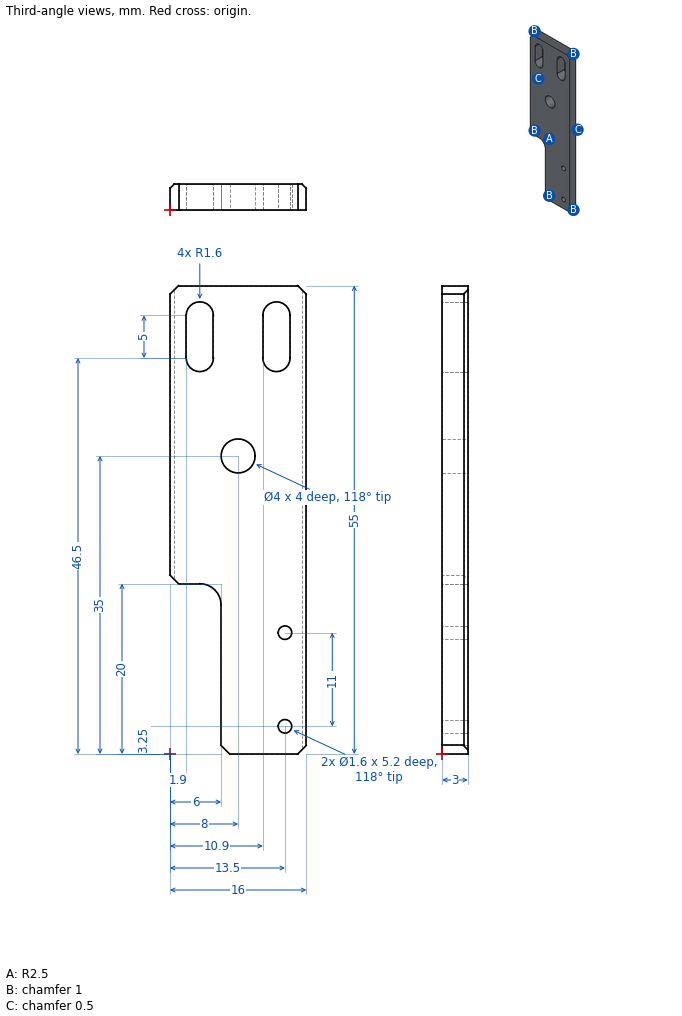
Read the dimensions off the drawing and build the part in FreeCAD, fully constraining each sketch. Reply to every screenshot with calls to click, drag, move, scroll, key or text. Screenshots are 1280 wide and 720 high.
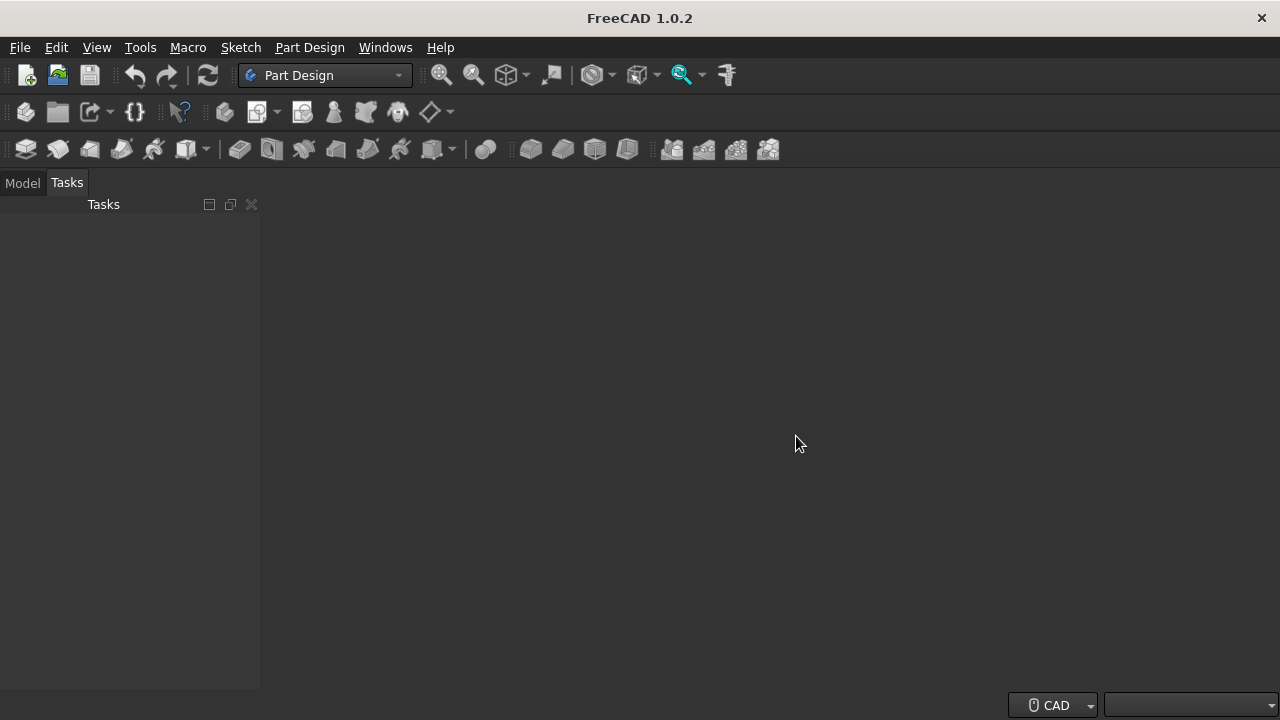
click(26, 76)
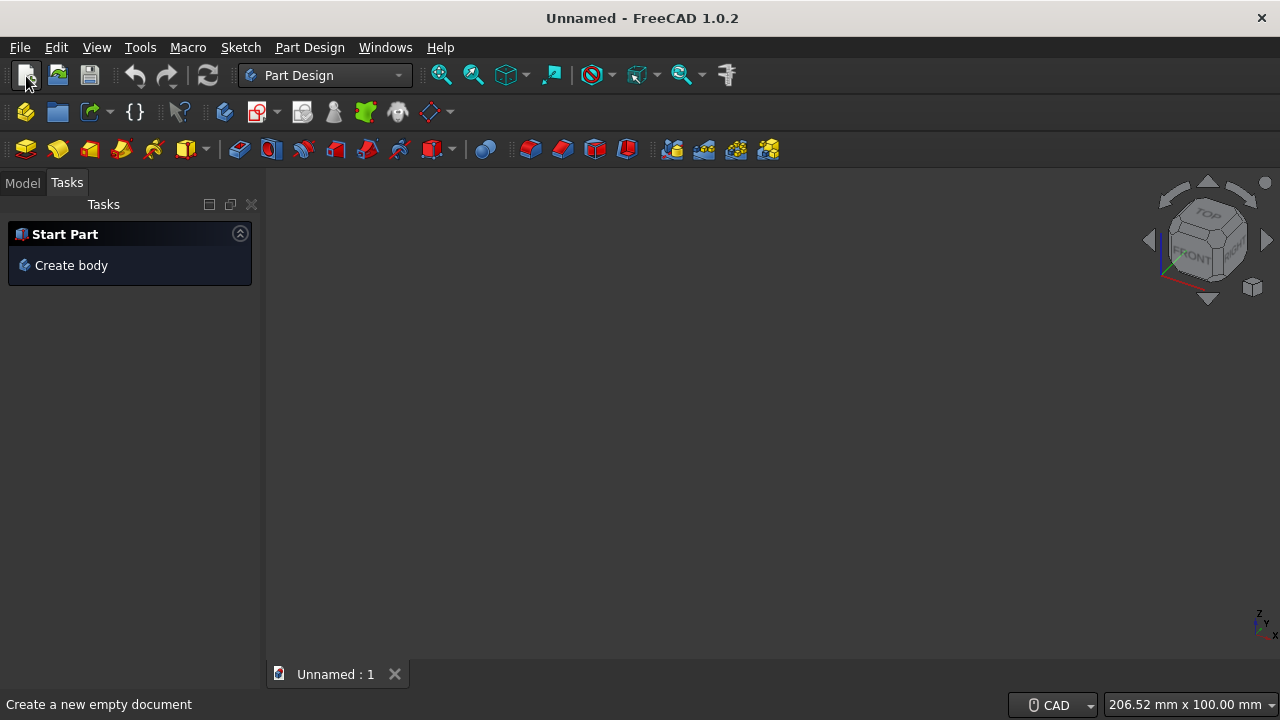
click(258, 112)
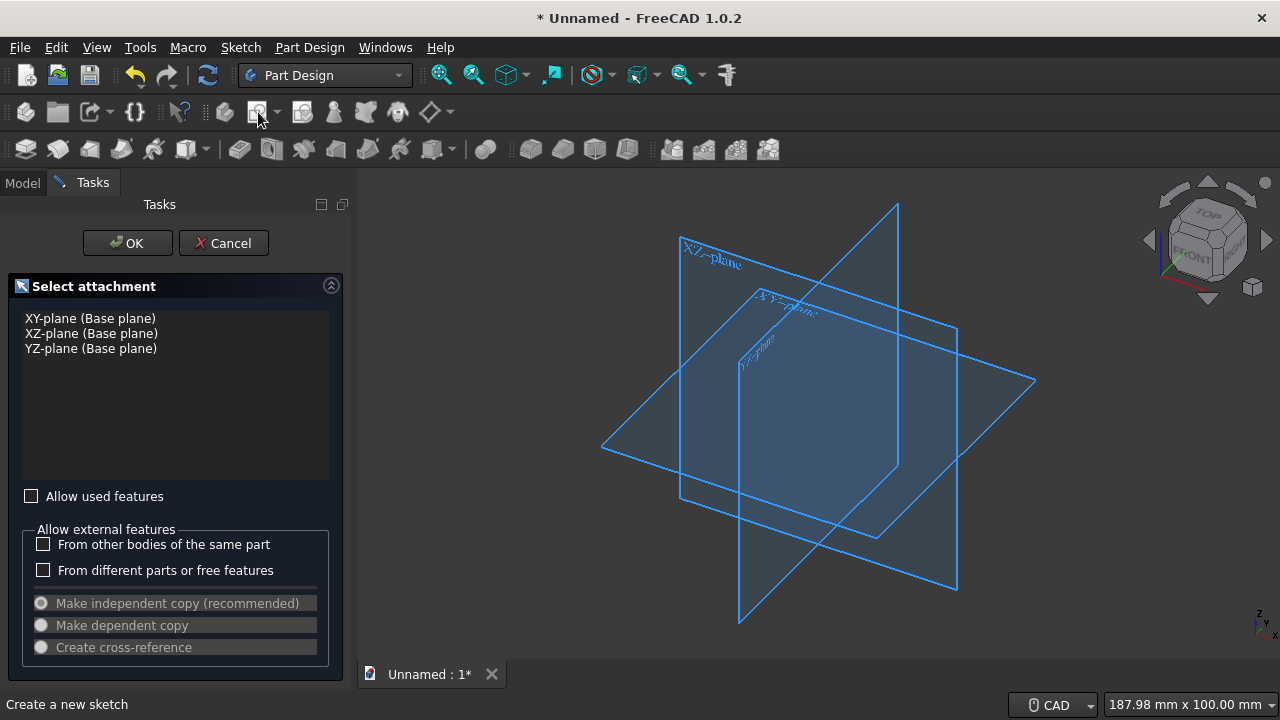
click(82, 334)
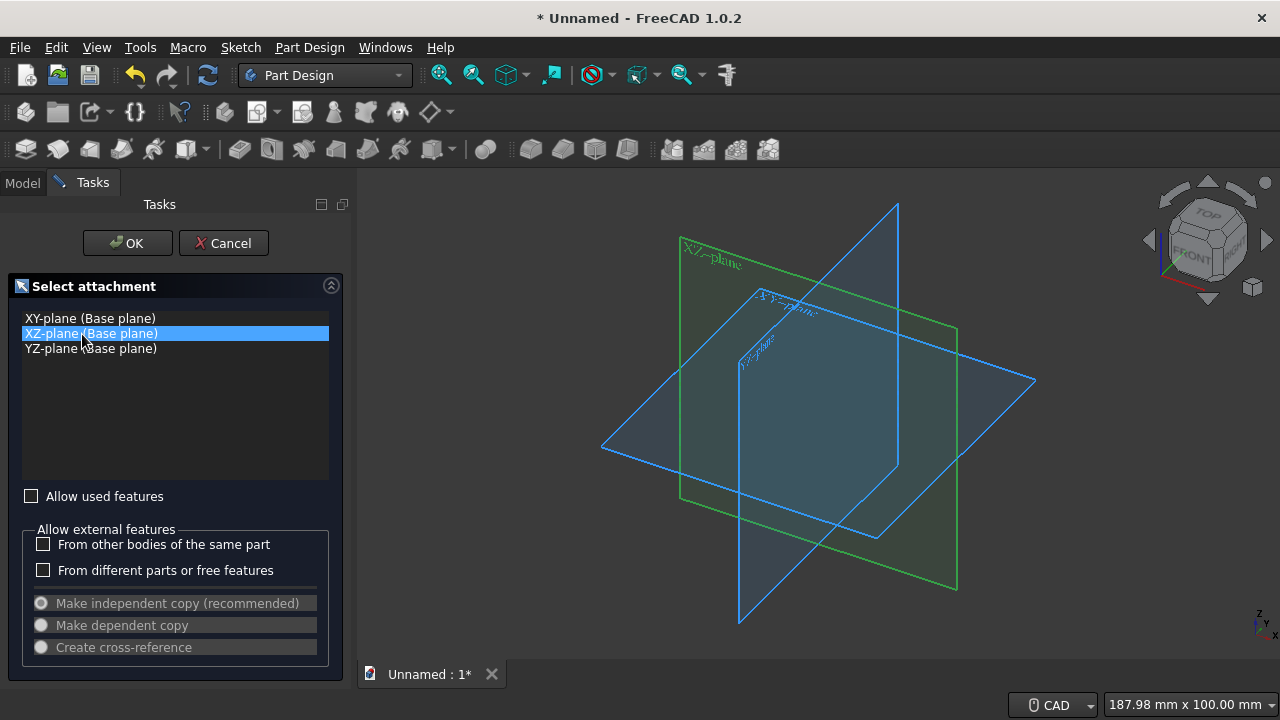
click(128, 243)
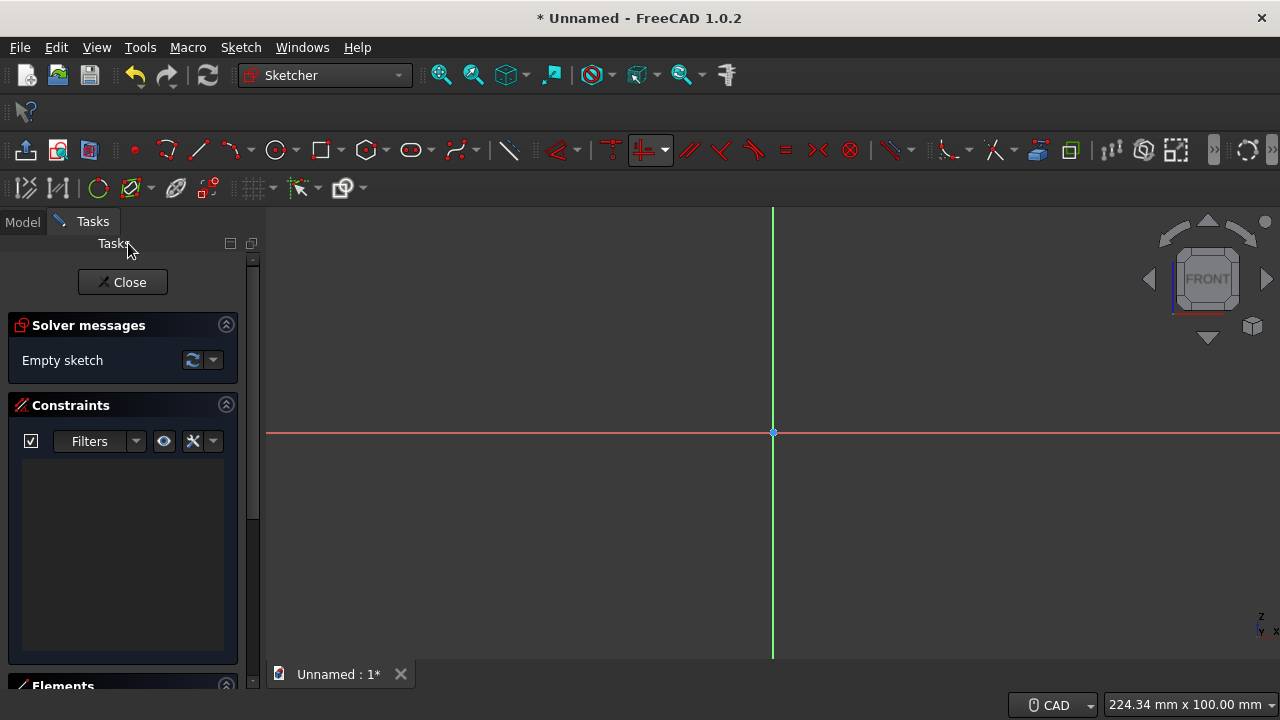
scroll(294, 631, down, 1)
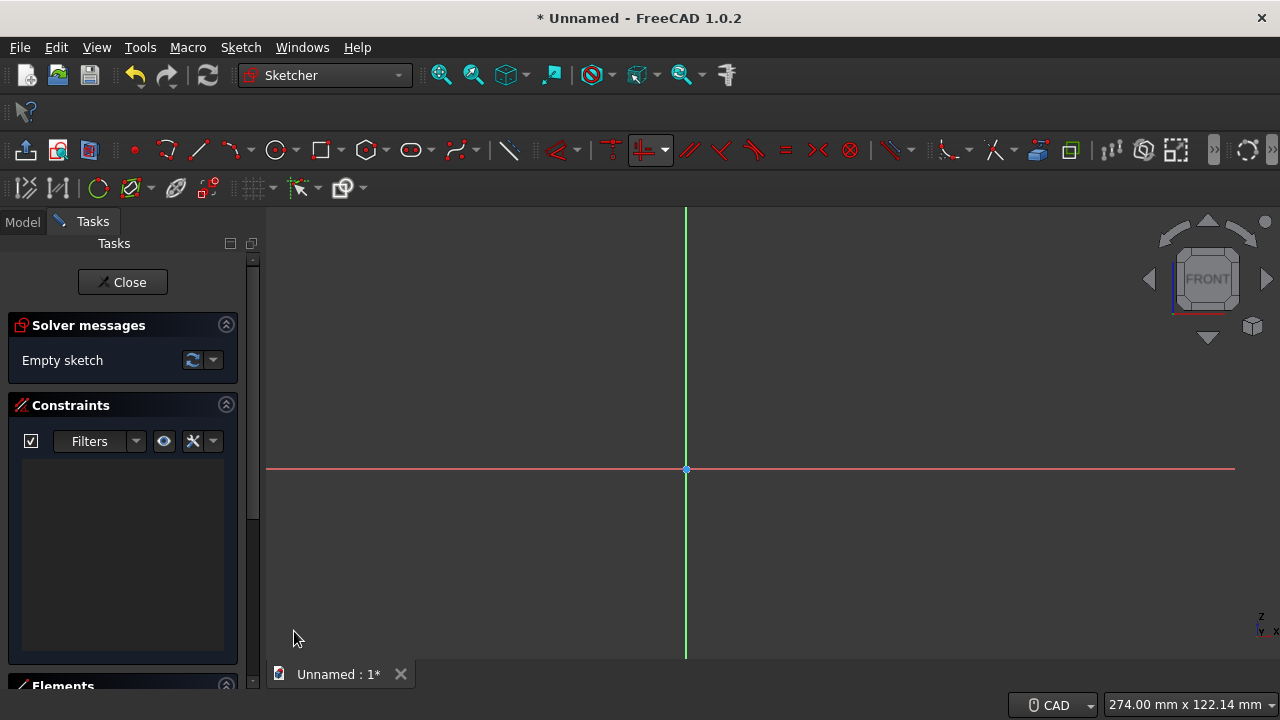
scroll(739, 235, up, 2)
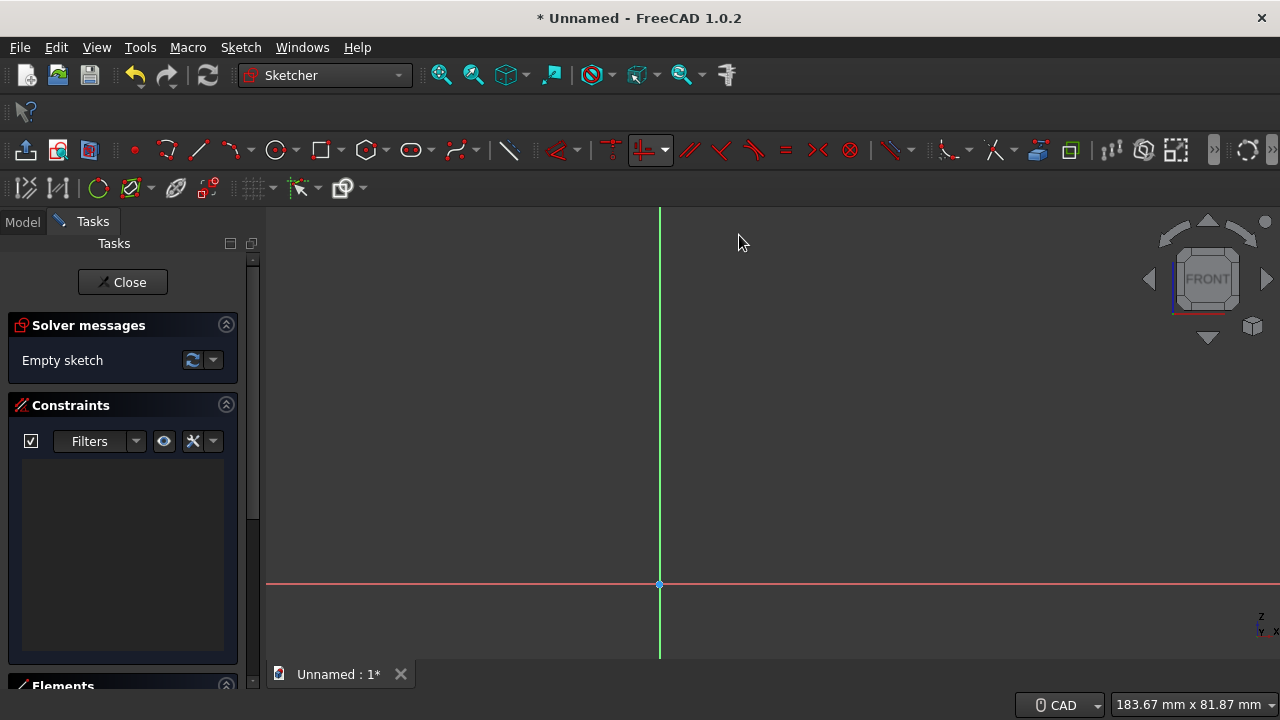
click(322, 150)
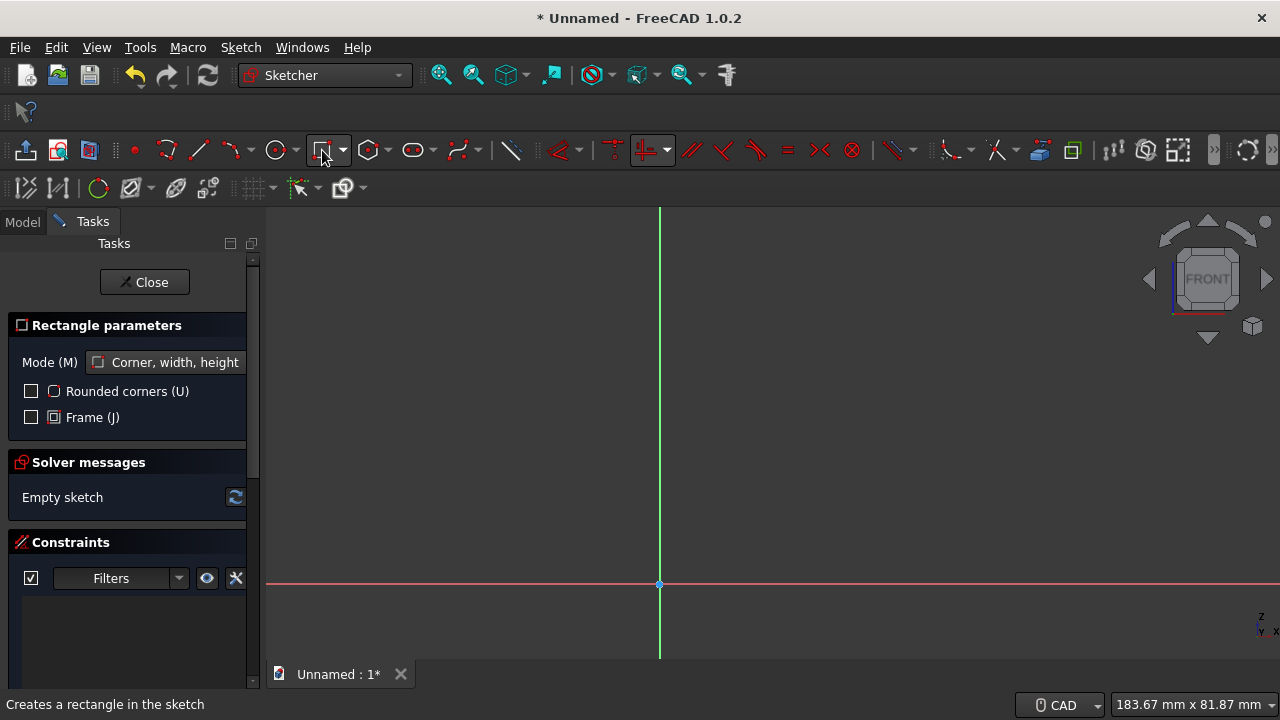
click(660, 584)
move(748, 281)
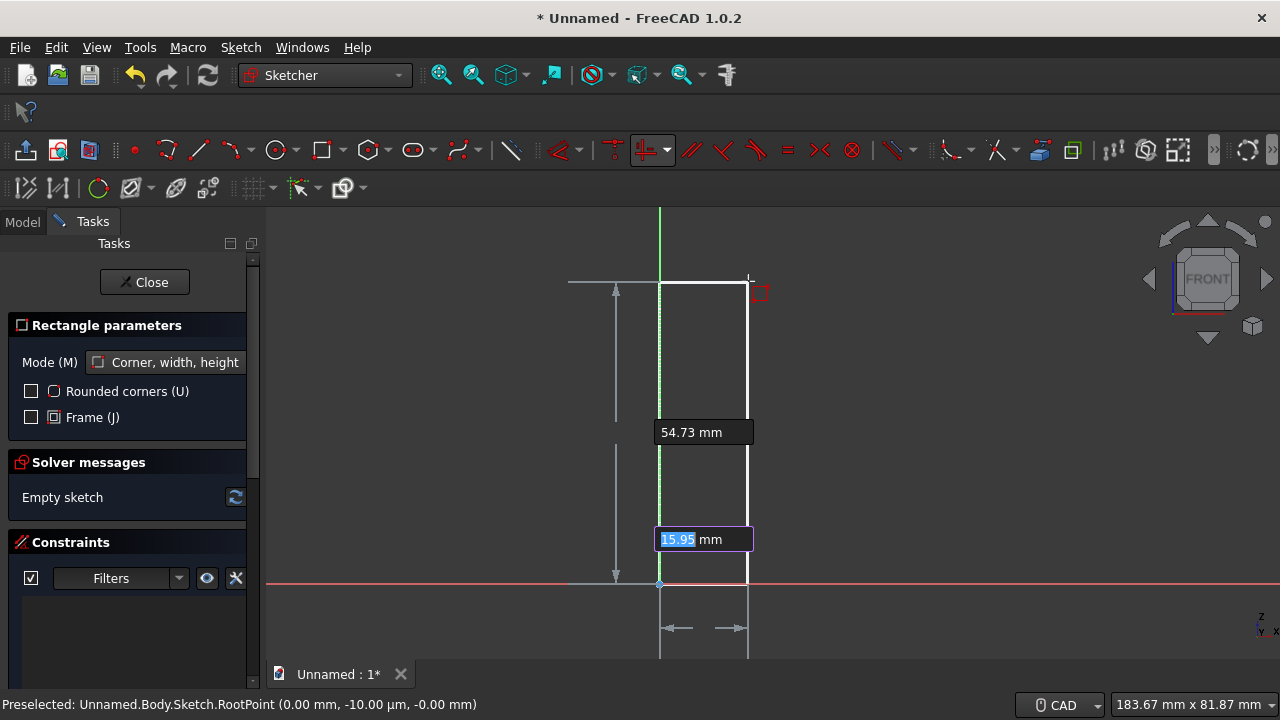
text(16)
key(Tab)
text(55)
key(Return)
key(Escape)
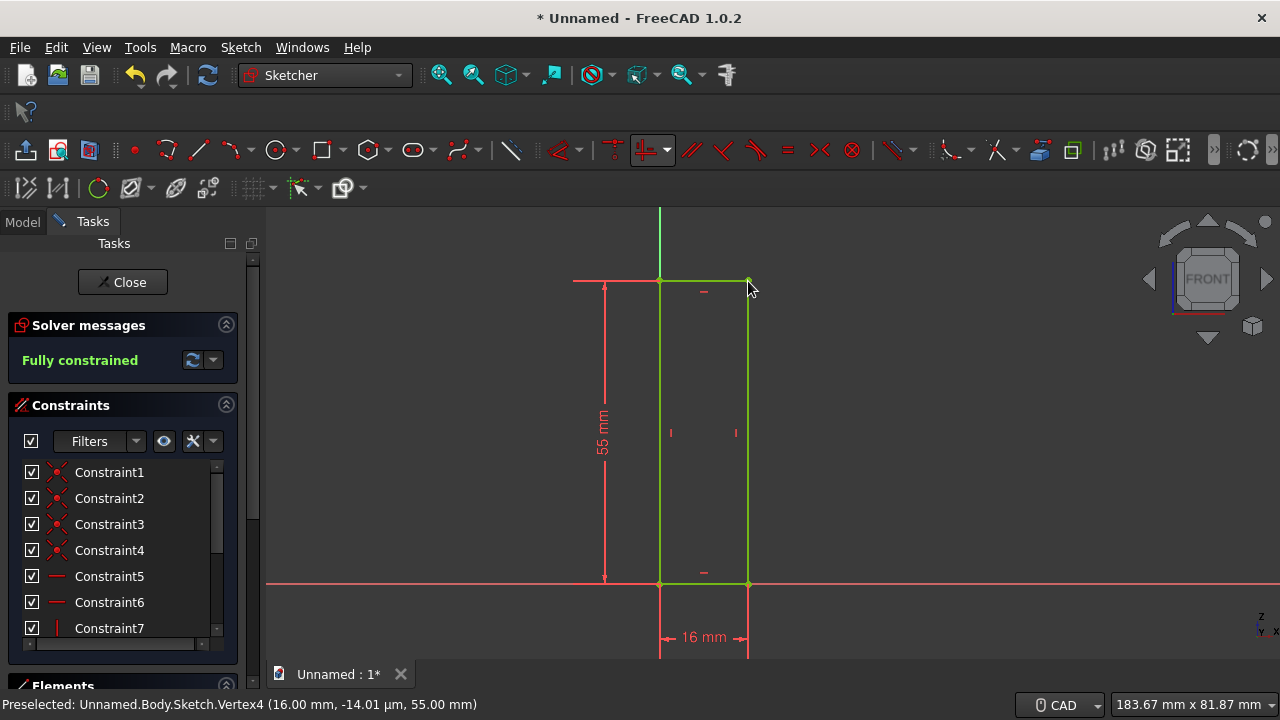
click(123, 282)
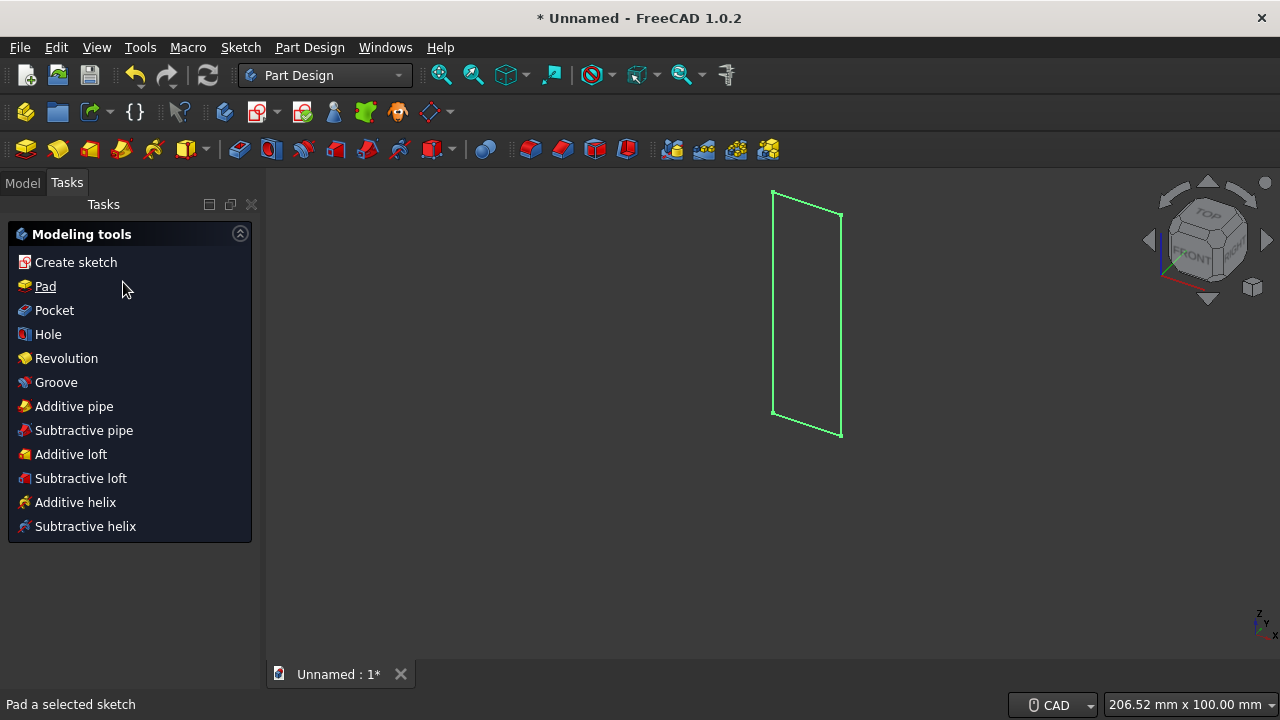
click(26, 150)